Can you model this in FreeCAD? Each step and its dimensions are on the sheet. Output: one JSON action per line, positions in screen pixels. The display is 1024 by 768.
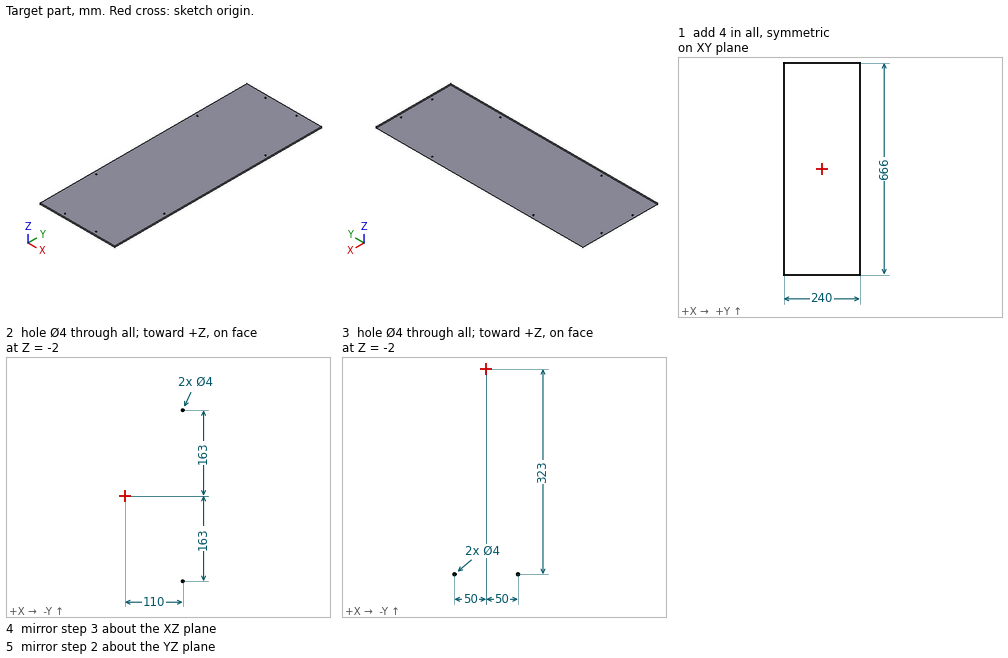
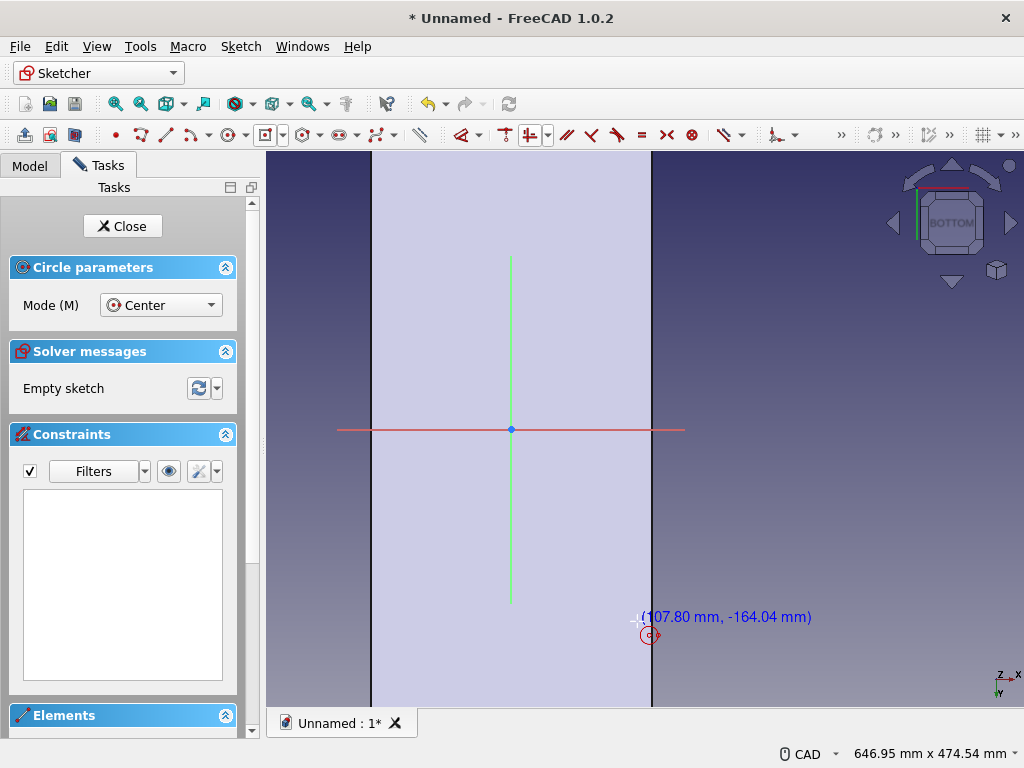
{"action": "left_click", "coordinate": [640, 621]}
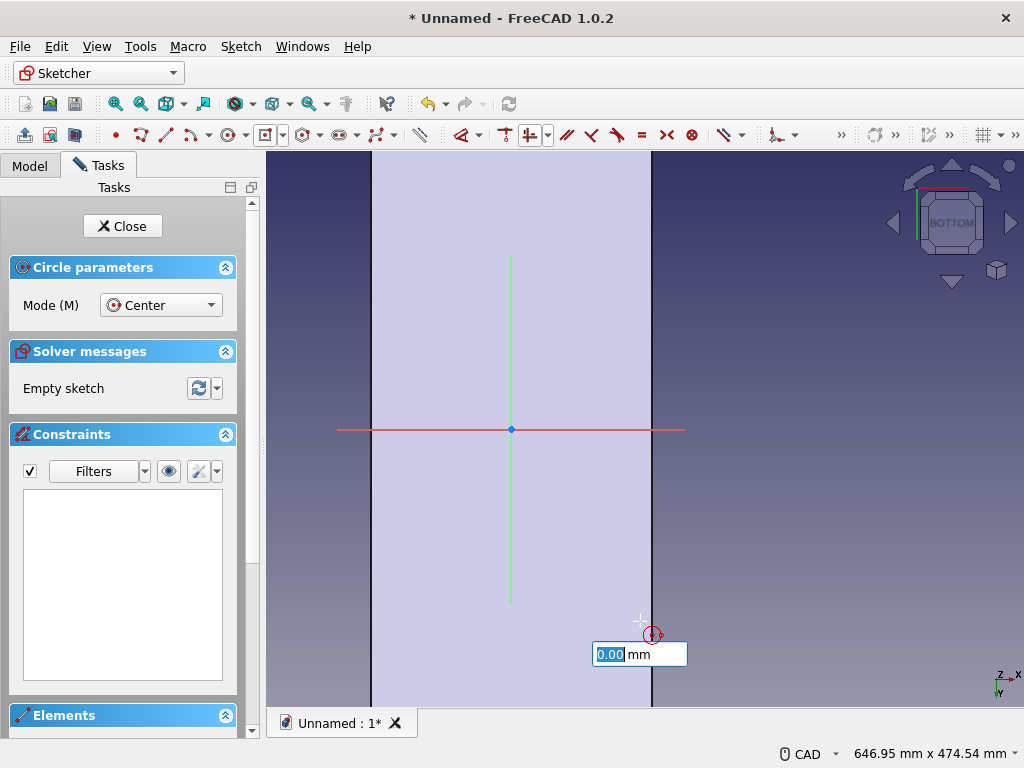
{"action": "scroll", "coordinate": [642, 619], "scroll_direction": "up", "scroll_amount": 10}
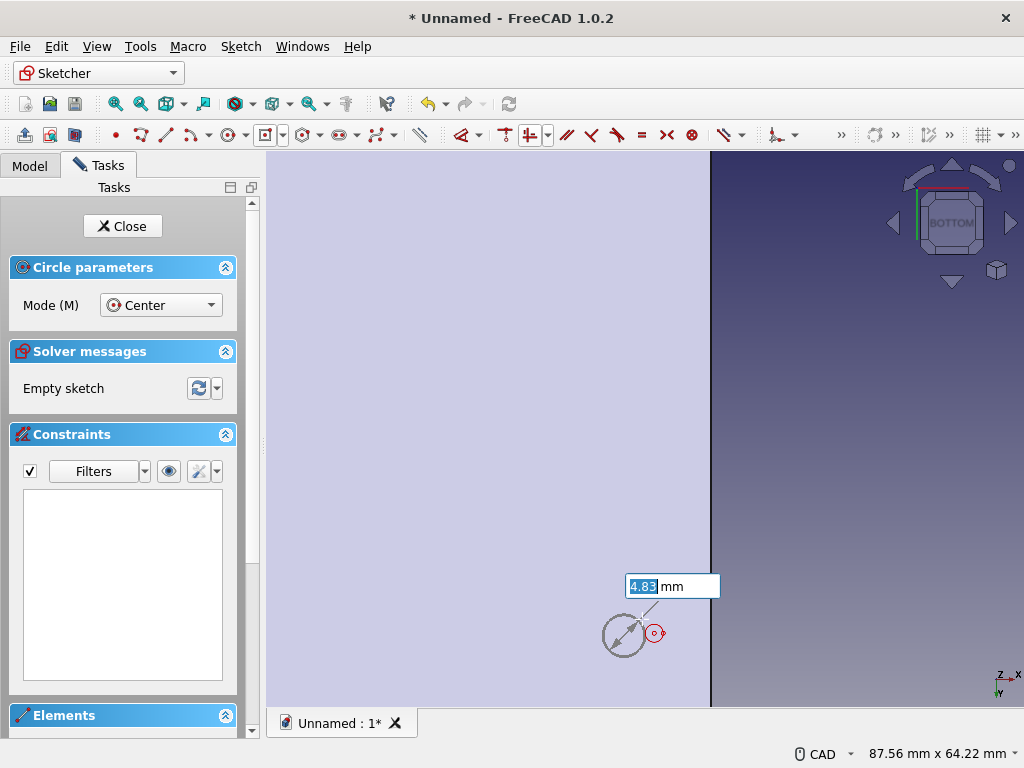
{"action": "left_click", "coordinate": [636, 614]}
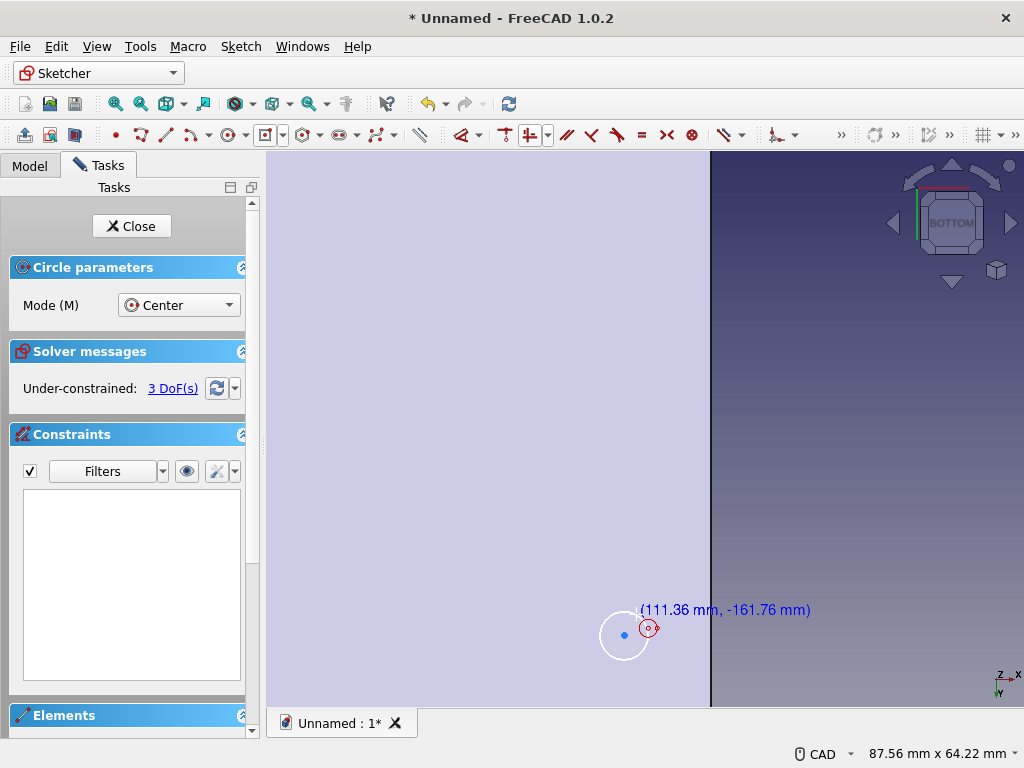
{"action": "scroll", "coordinate": [642, 619], "scroll_direction": "down", "scroll_amount": 10}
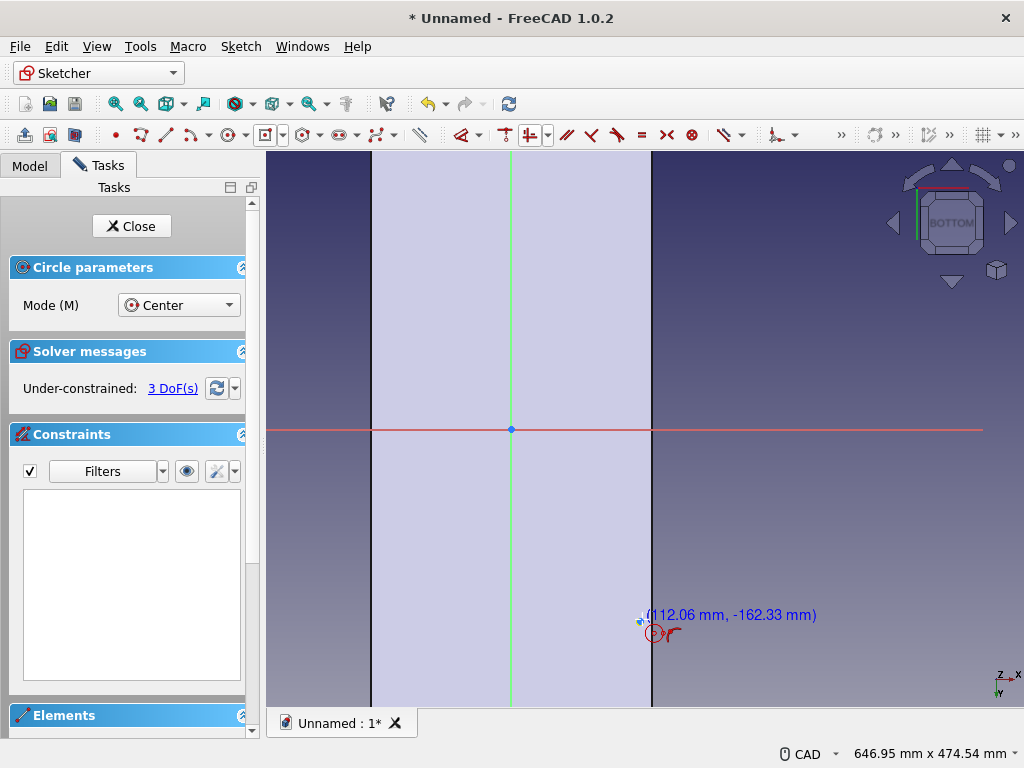
{"action": "scroll", "coordinate": [640, 239], "scroll_direction": "up", "scroll_amount": 12}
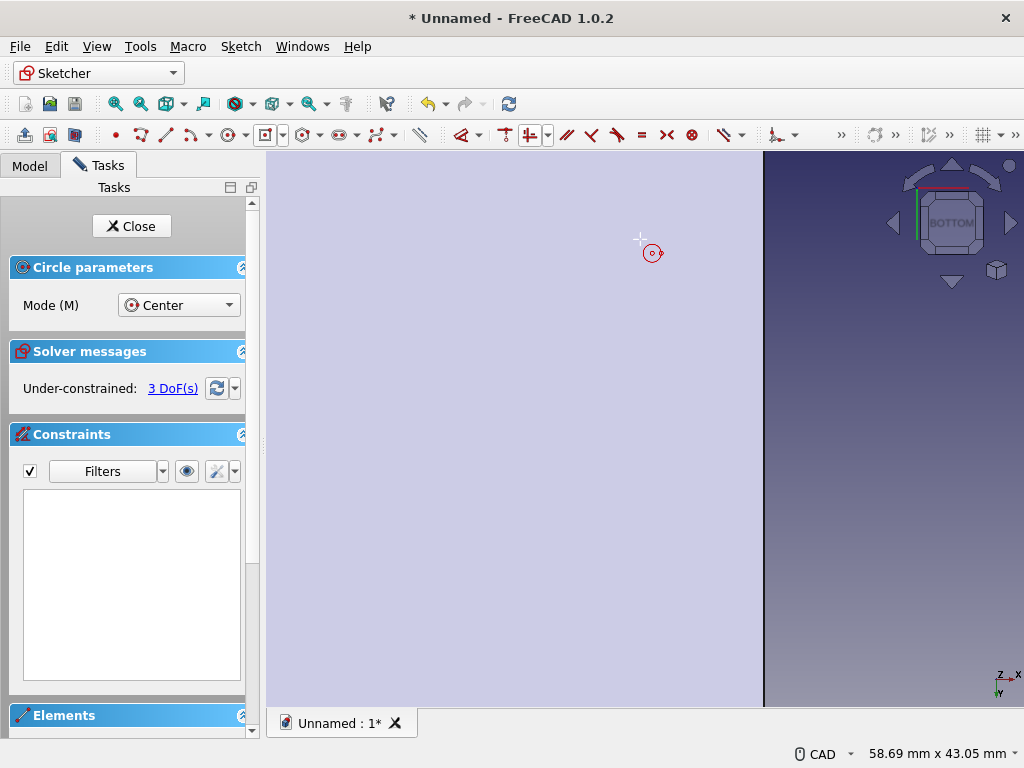
{"action": "scroll", "coordinate": [640, 238], "scroll_direction": "down", "scroll_amount": 12}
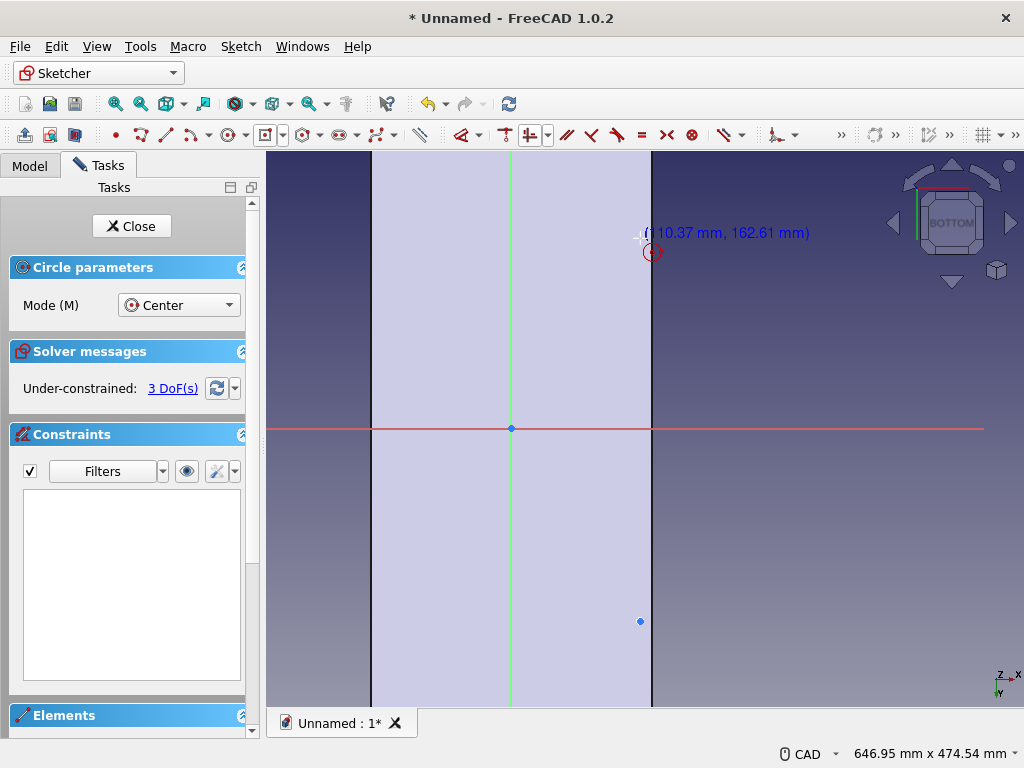
{"action": "left_click", "coordinate": [640, 238]}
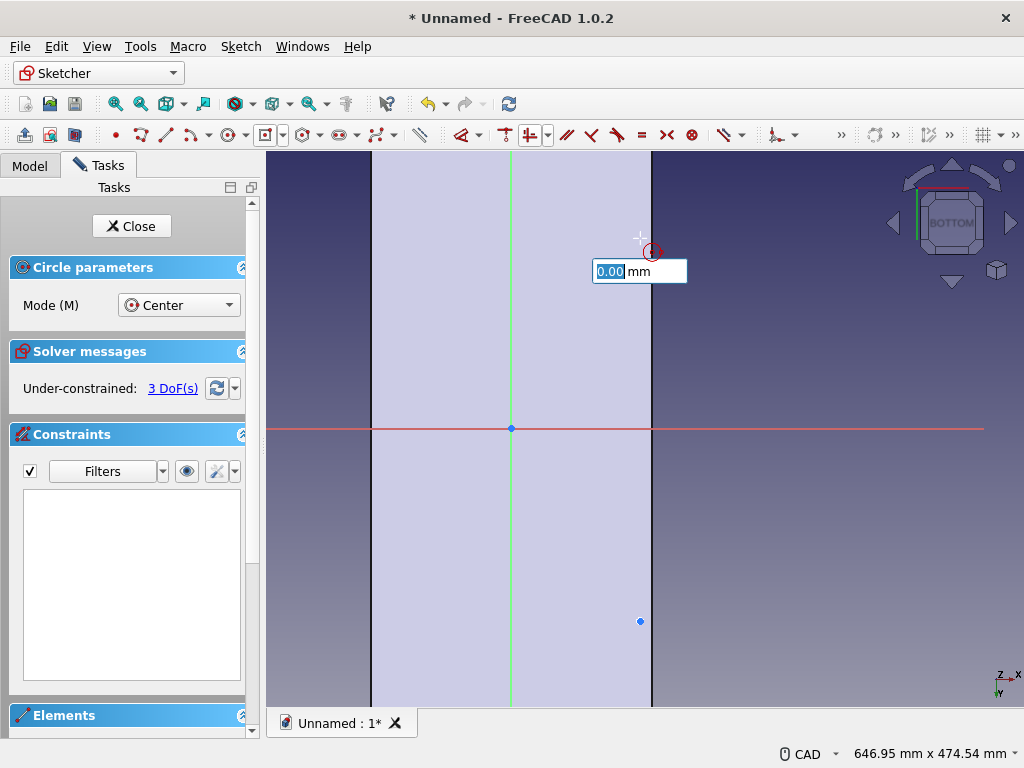
{"action": "scroll", "coordinate": [642, 236], "scroll_direction": "up", "scroll_amount": 10}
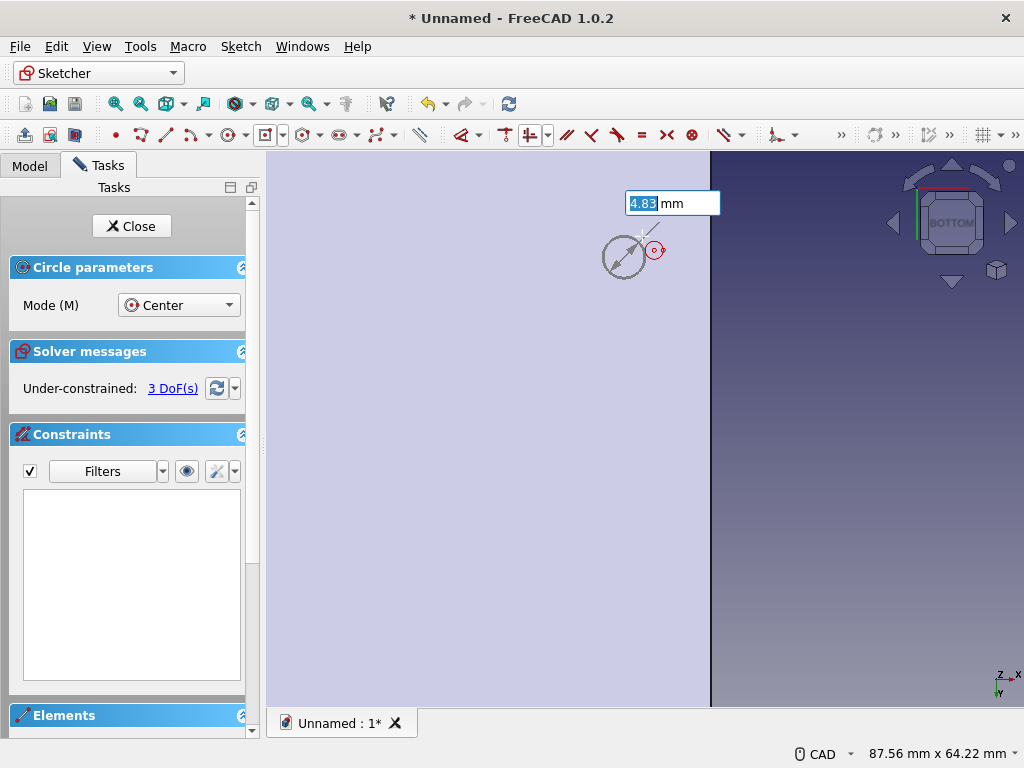
{"action": "left_click", "coordinate": [636, 236]}
{"action": "key", "text": "Escape"}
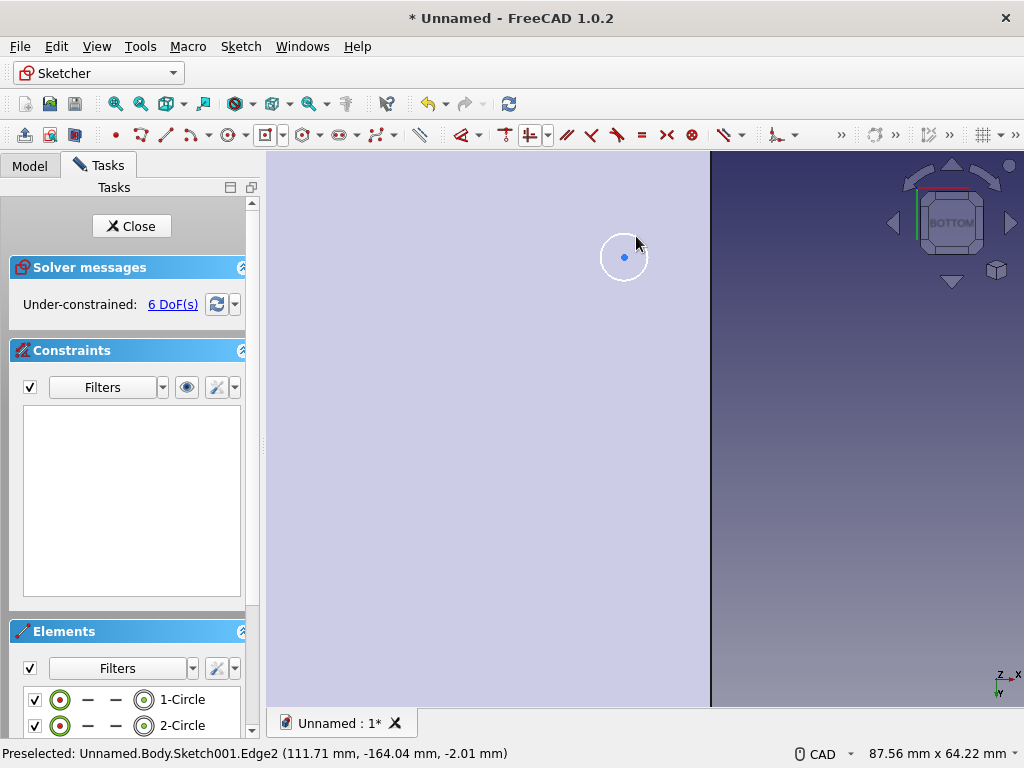
{"action": "scroll", "coordinate": [642, 236], "scroll_direction": "down", "scroll_amount": 10}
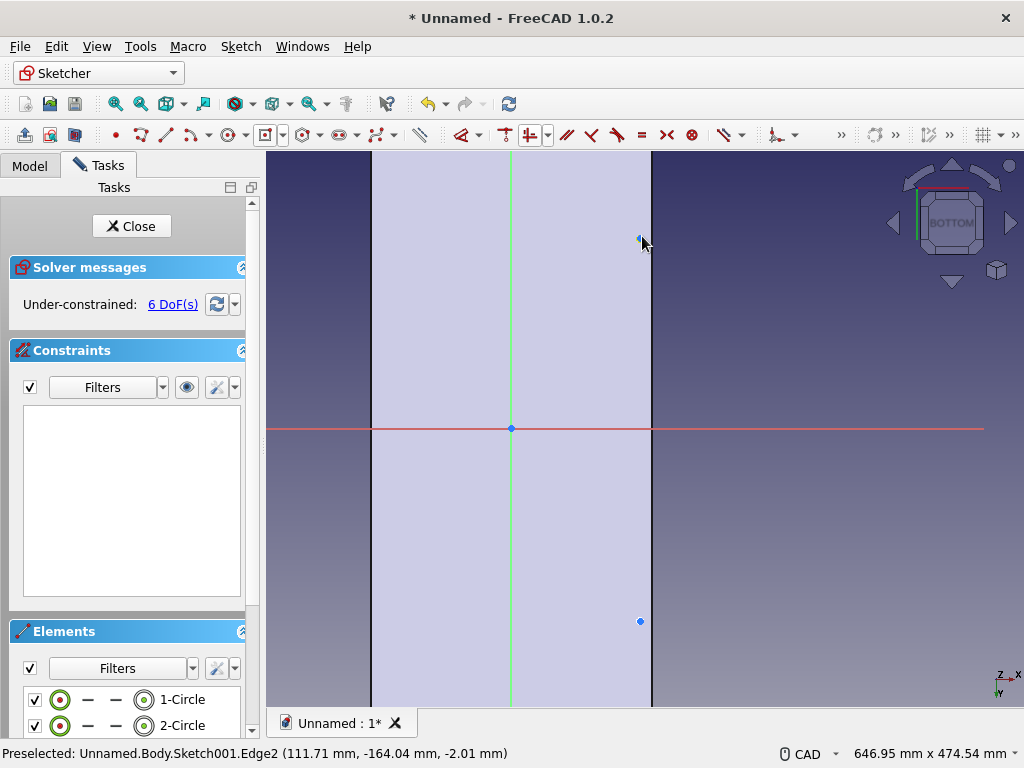
{"action": "scroll", "coordinate": [642, 619], "scroll_direction": "up", "scroll_amount": 8}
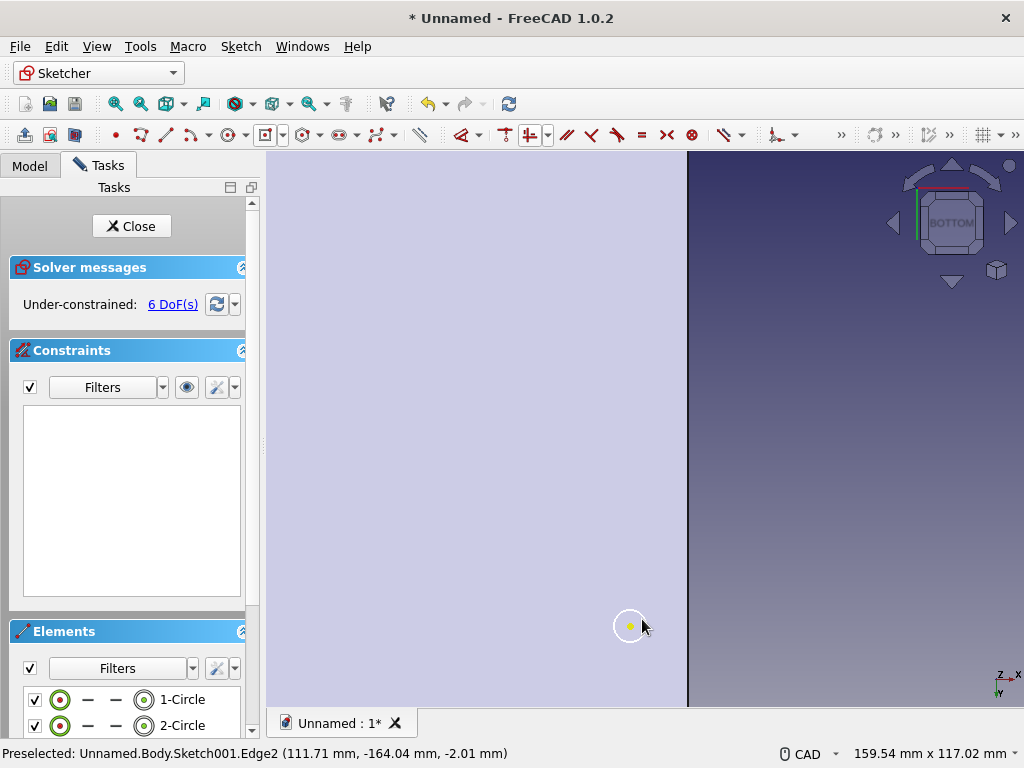
{"action": "left_click", "coordinate": [641, 615]}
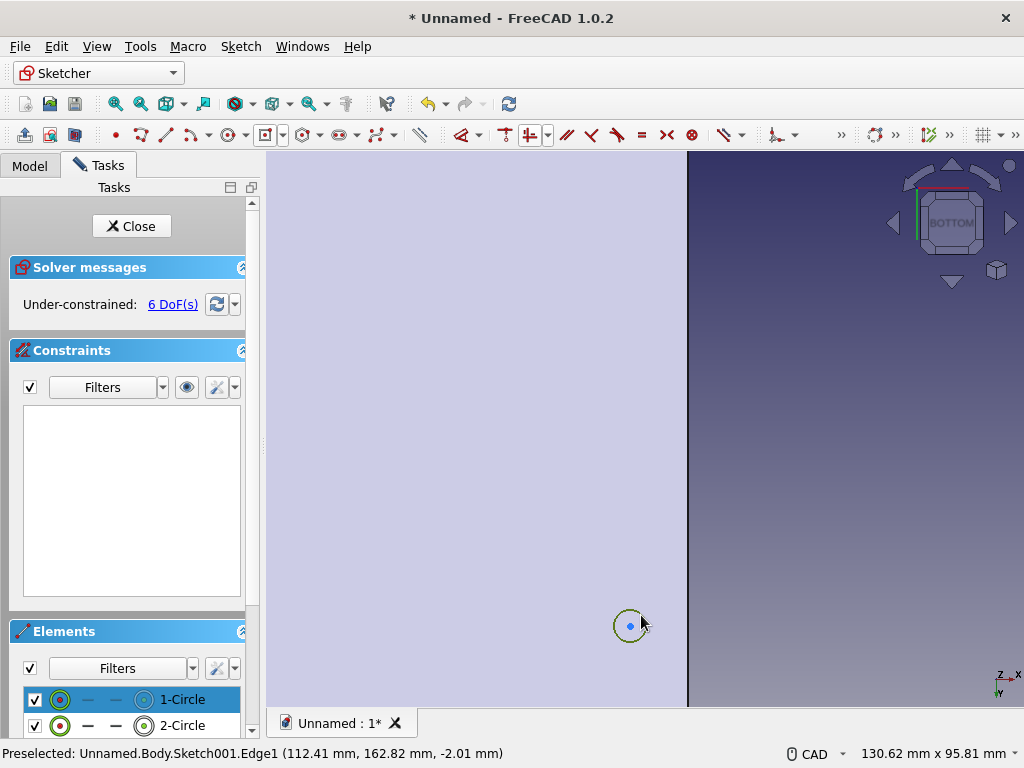
{"action": "scroll", "coordinate": [642, 620], "scroll_direction": "down", "scroll_amount": 8}